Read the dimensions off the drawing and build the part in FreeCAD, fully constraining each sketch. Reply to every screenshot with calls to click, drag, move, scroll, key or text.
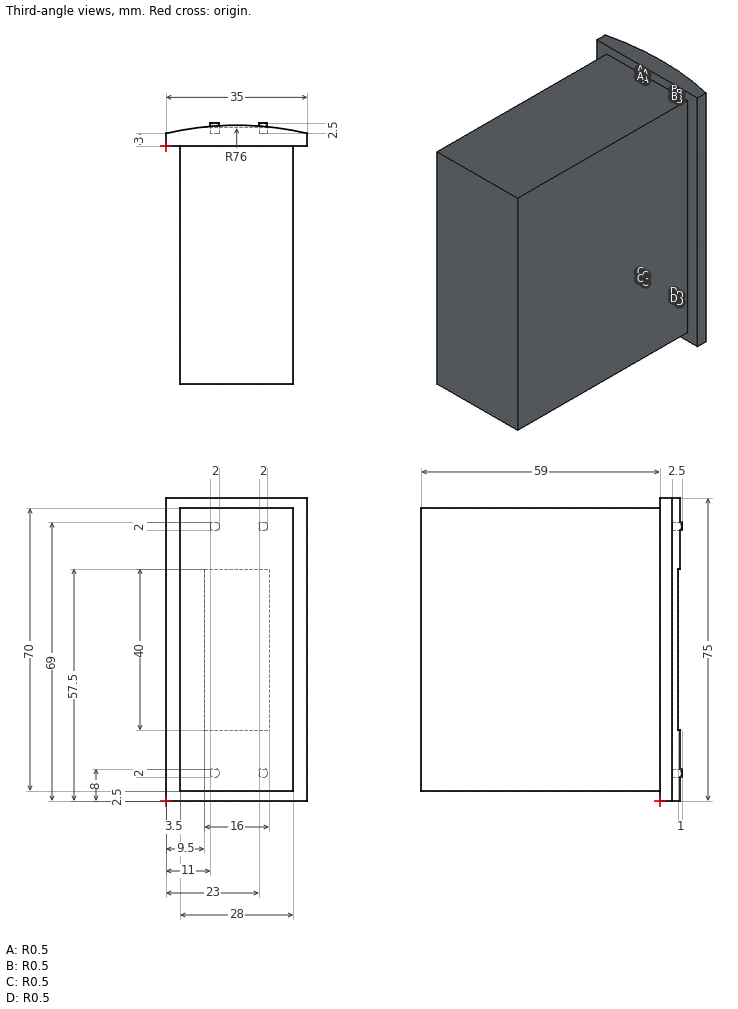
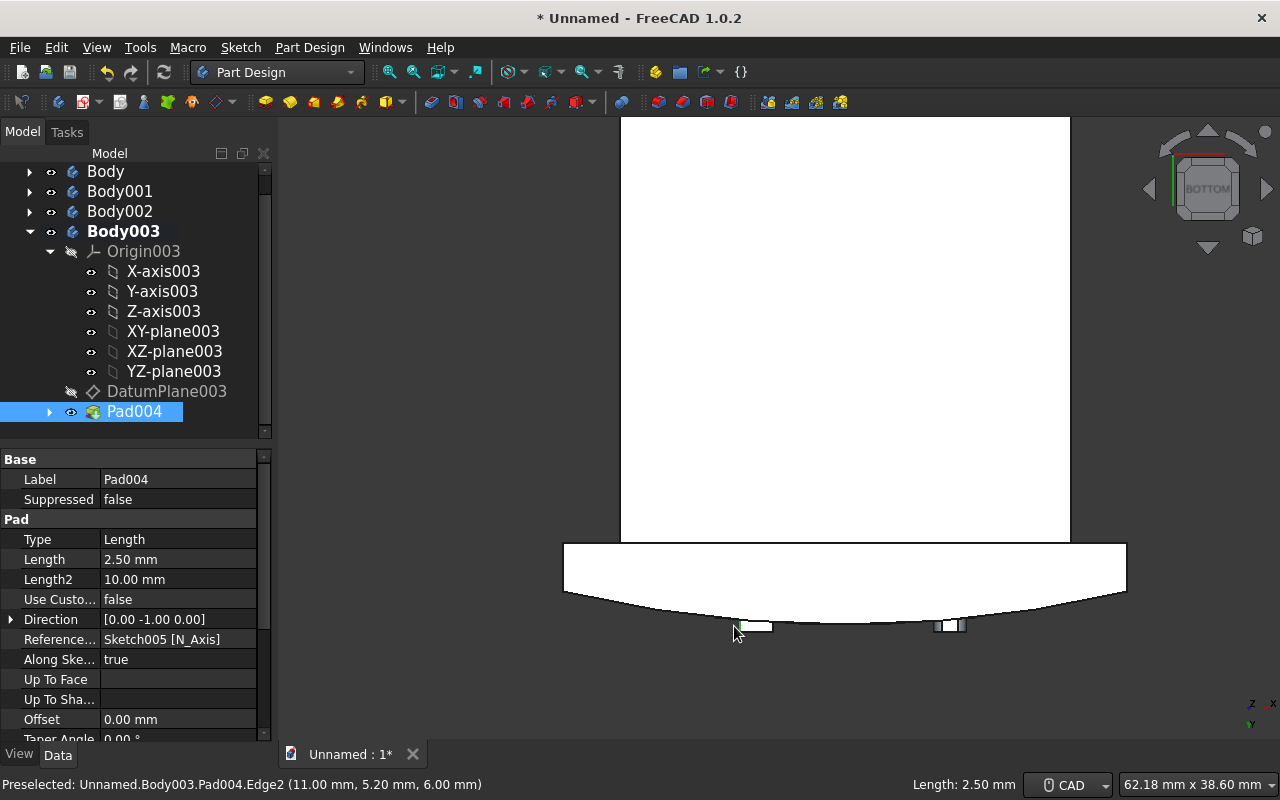
key(v)
key(f)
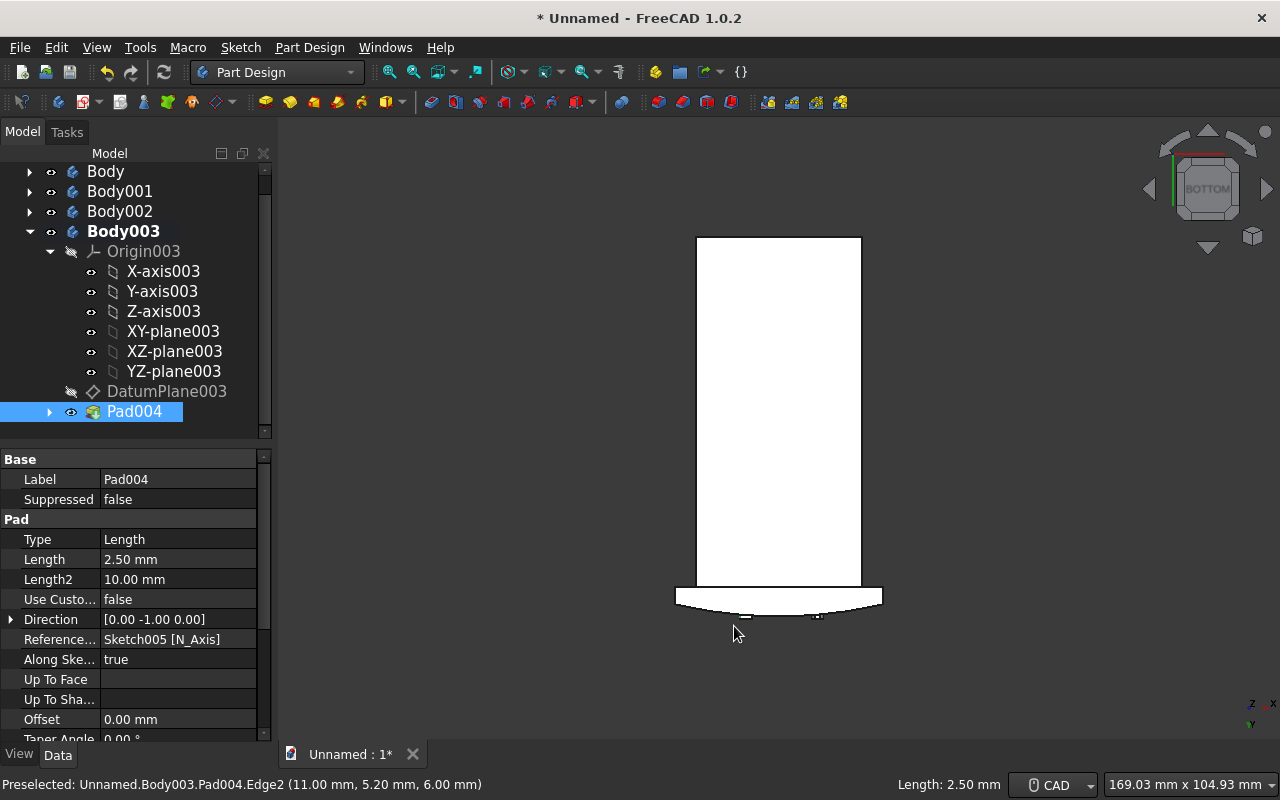
key(4)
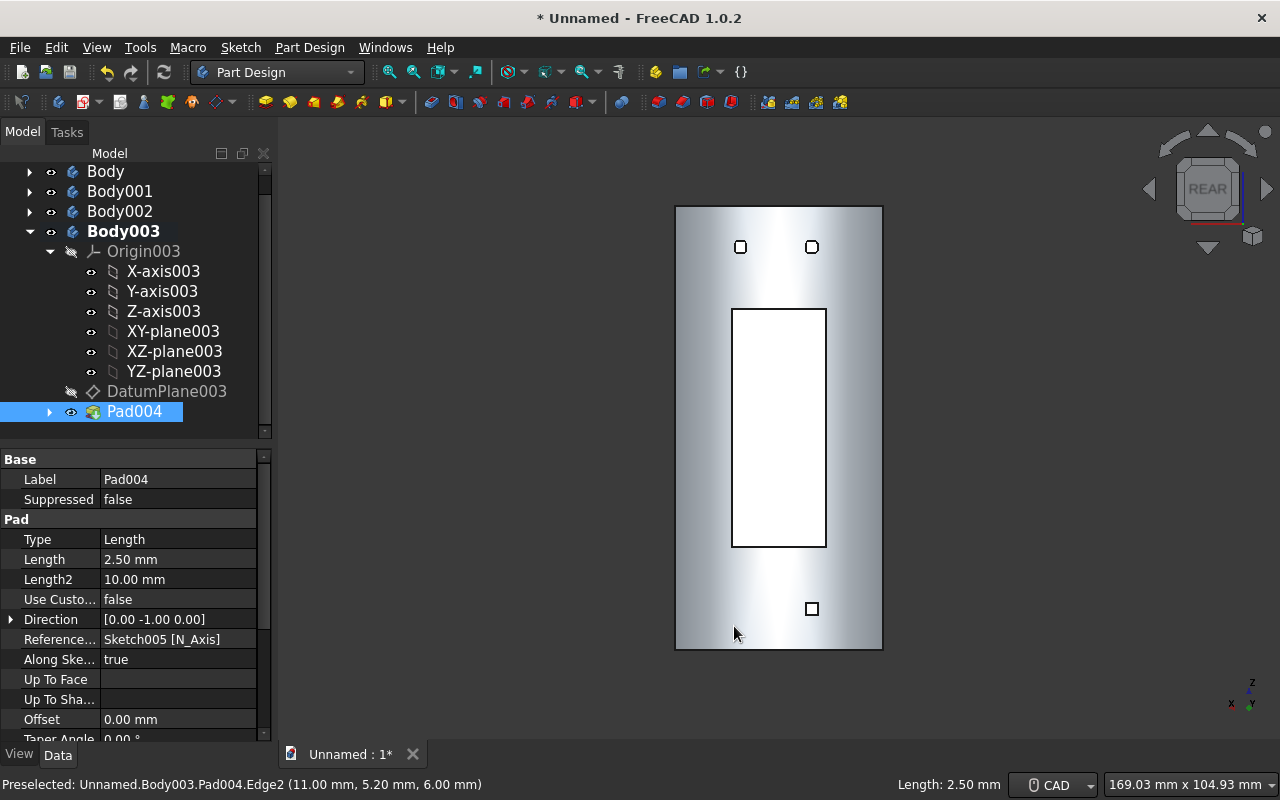
key(v)
key(f)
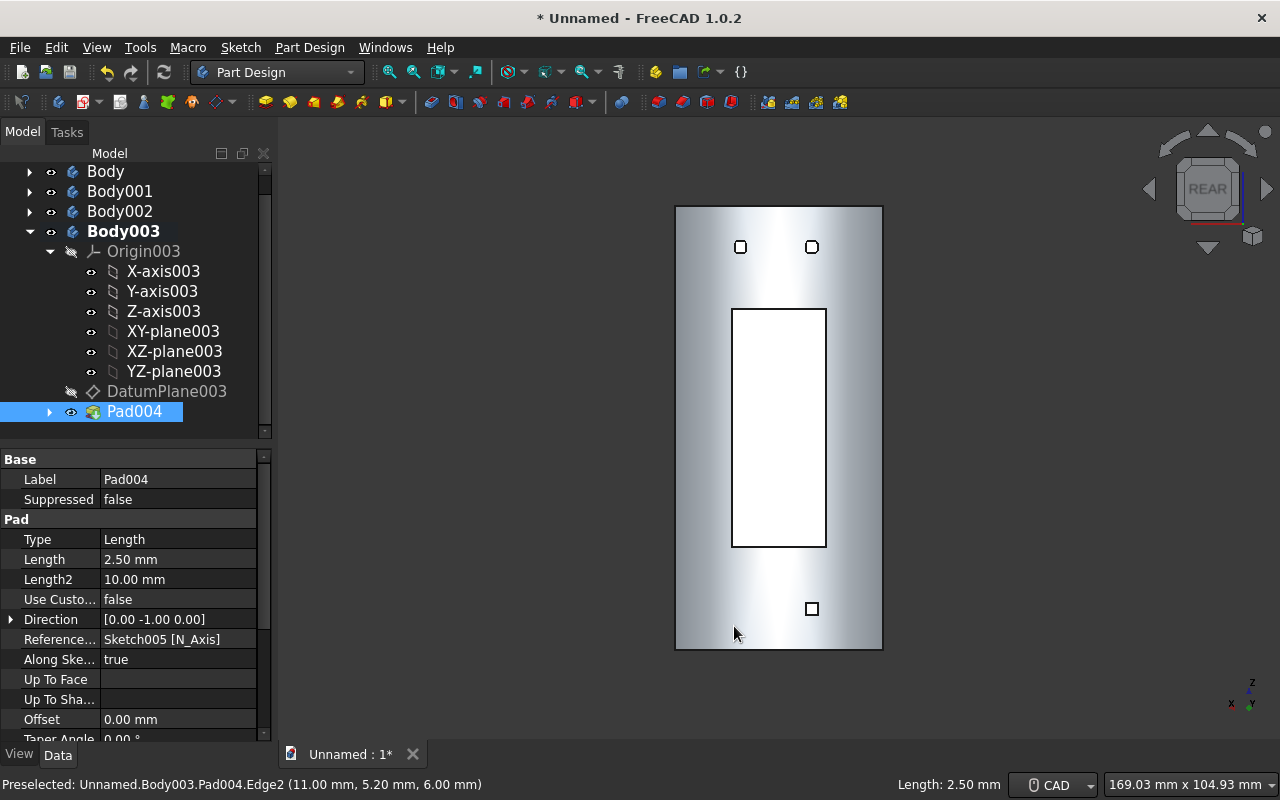
scroll(818, 602, up, 5)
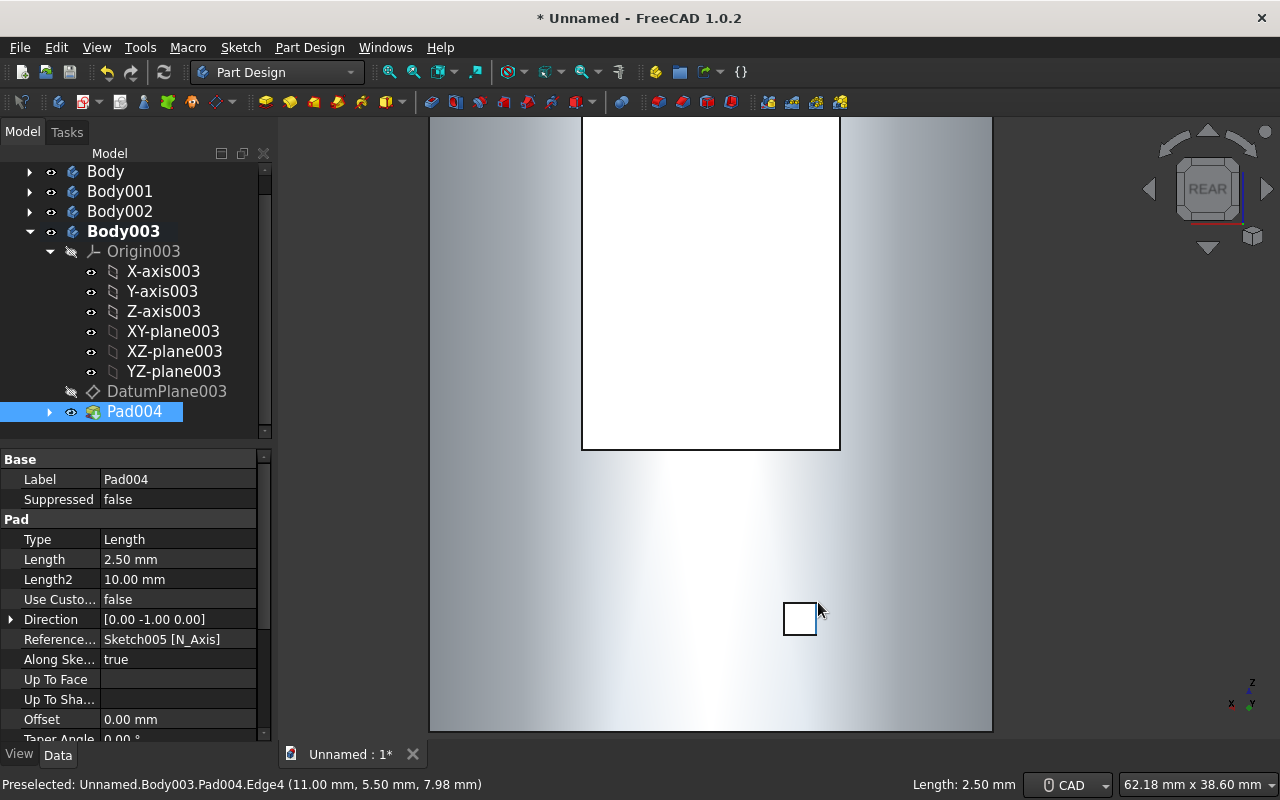
key(v)
key(f)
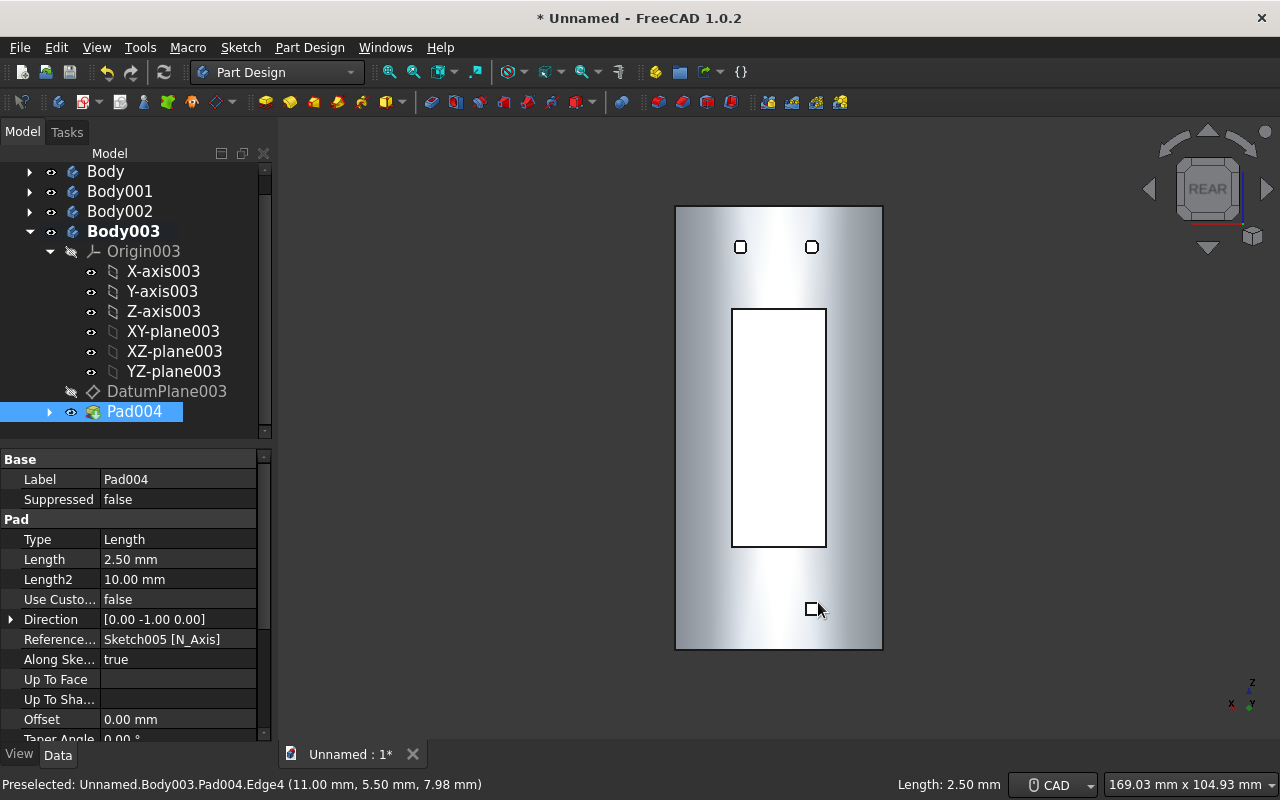
key(6)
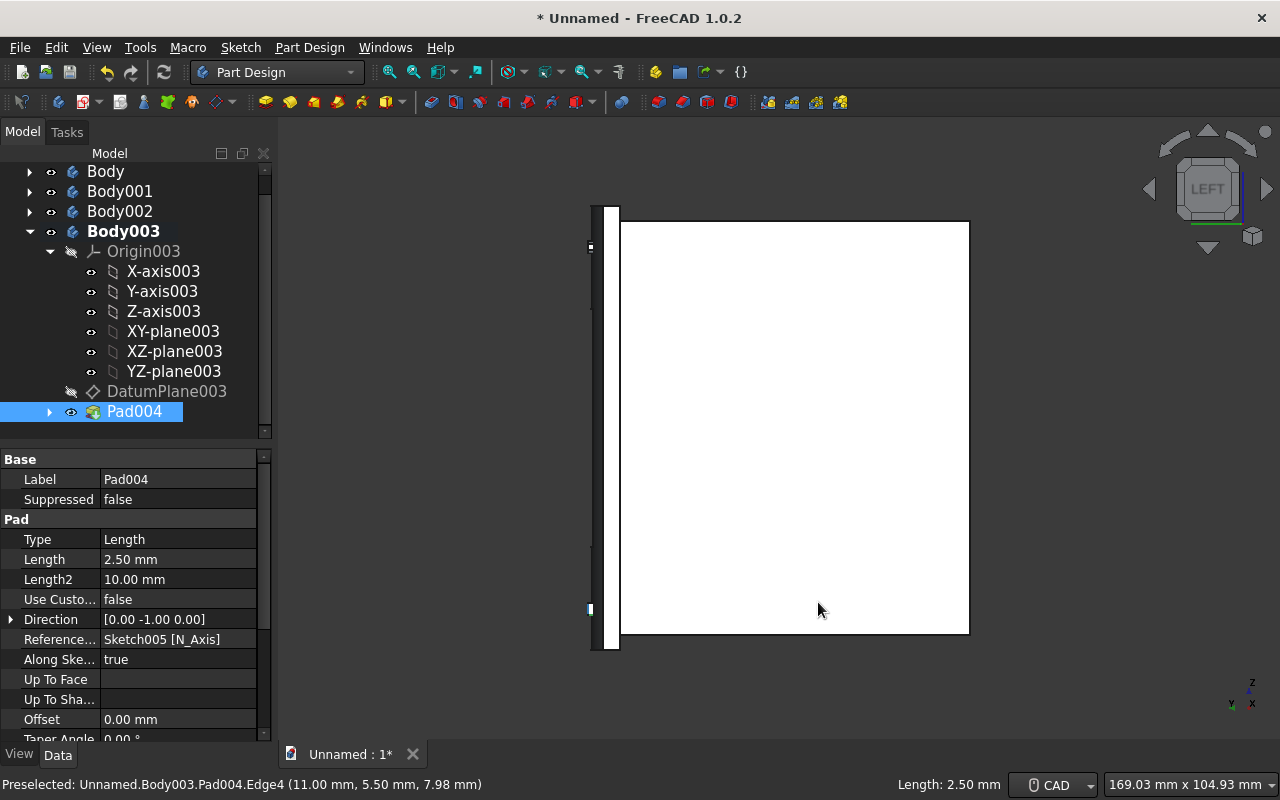
click(390, 72)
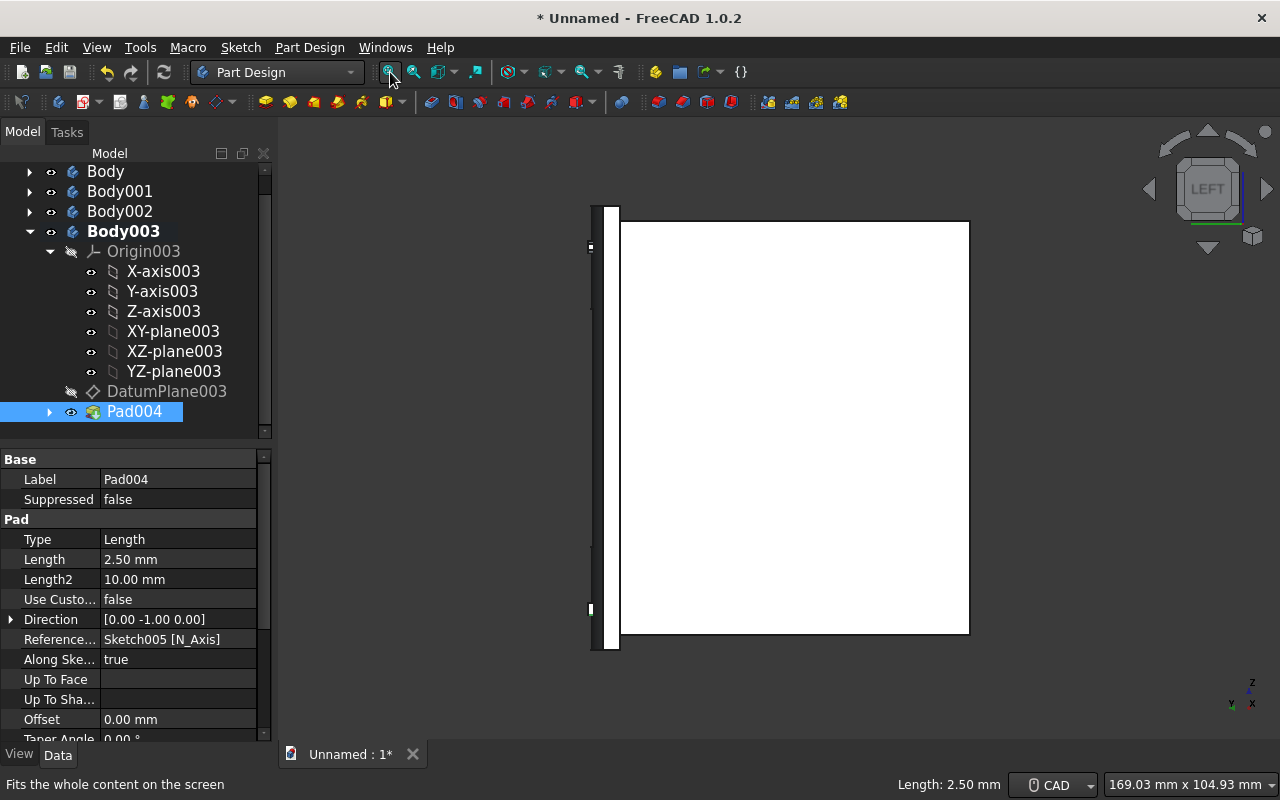
scroll(595, 602, up, 5)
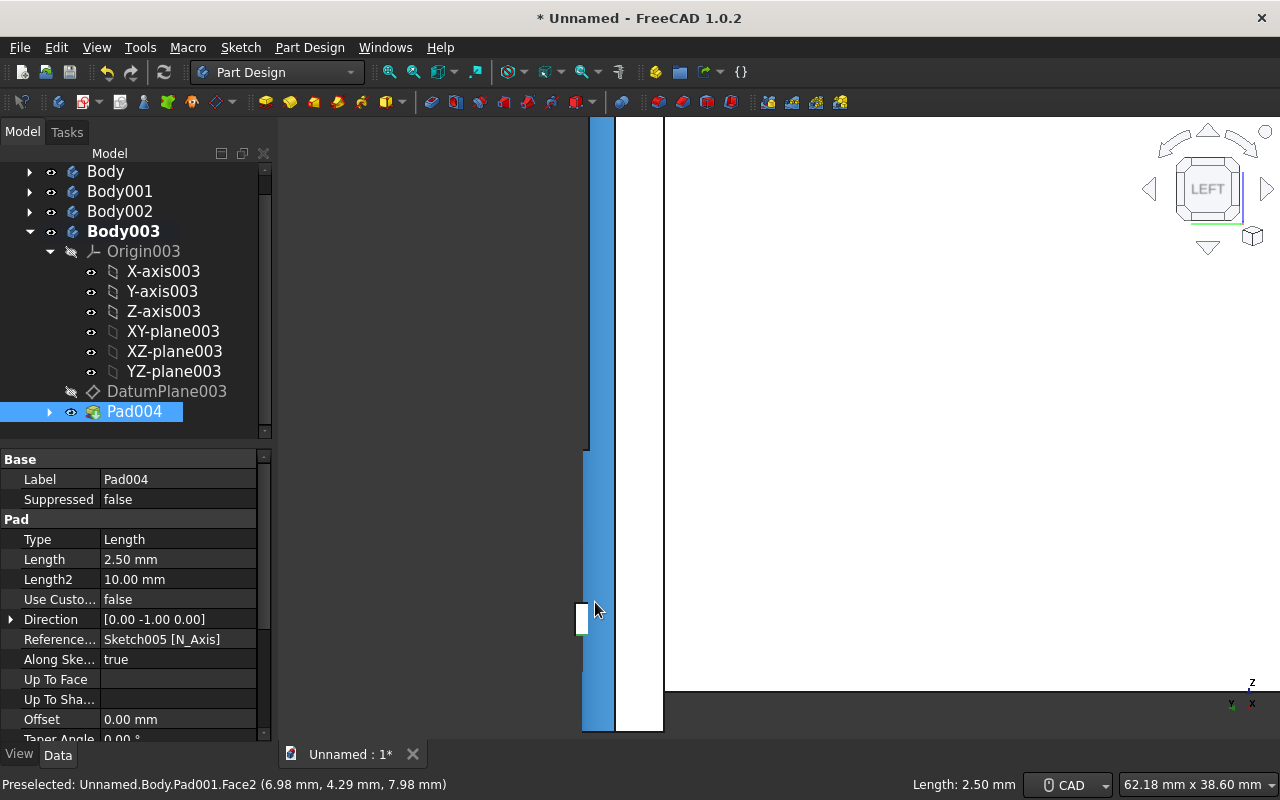
click(583, 602, ctrl)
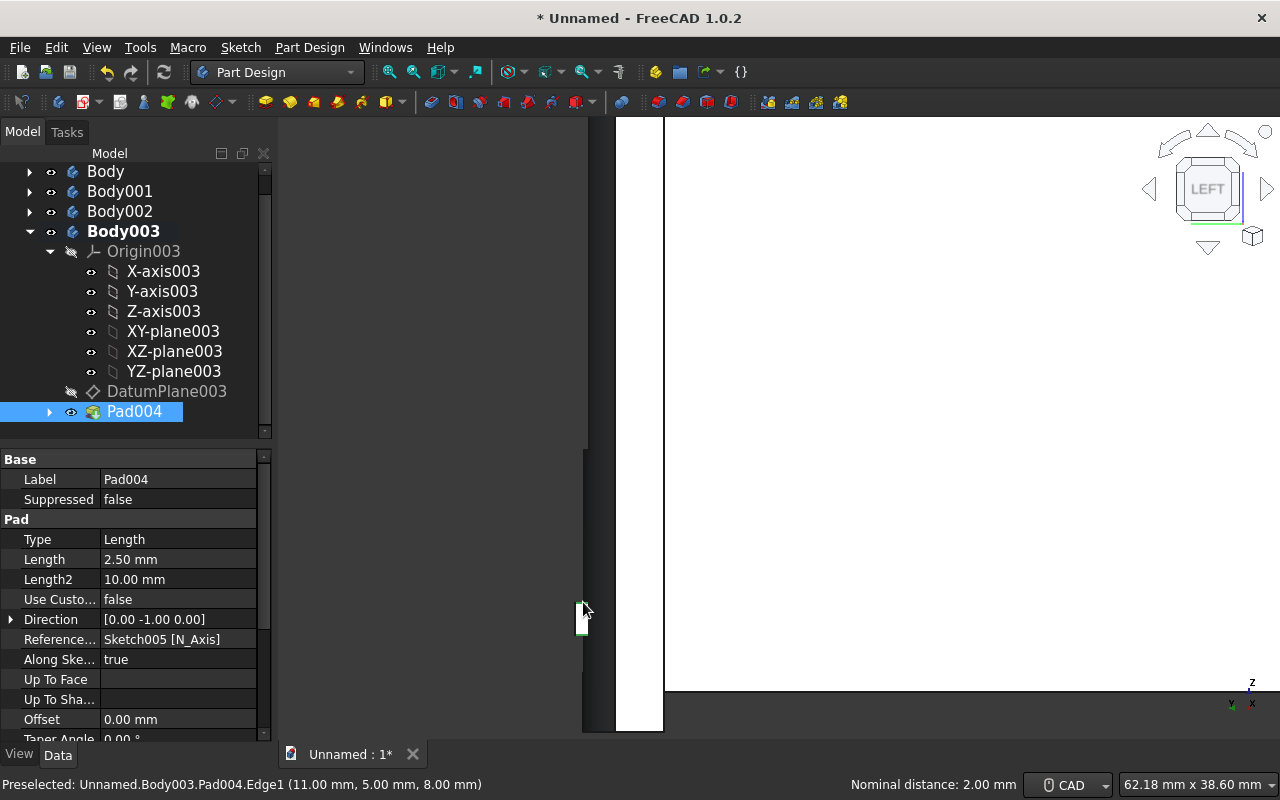
key(v)
key(f)